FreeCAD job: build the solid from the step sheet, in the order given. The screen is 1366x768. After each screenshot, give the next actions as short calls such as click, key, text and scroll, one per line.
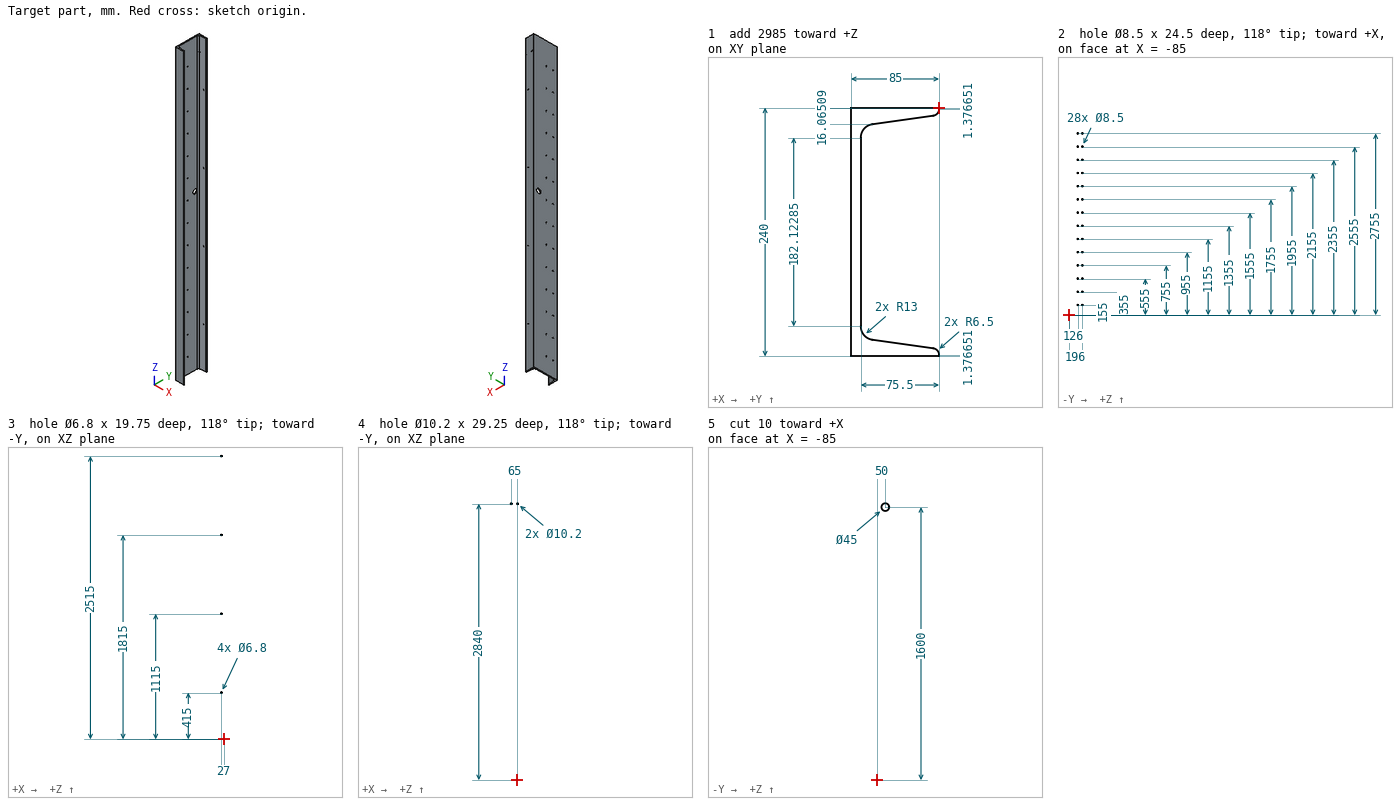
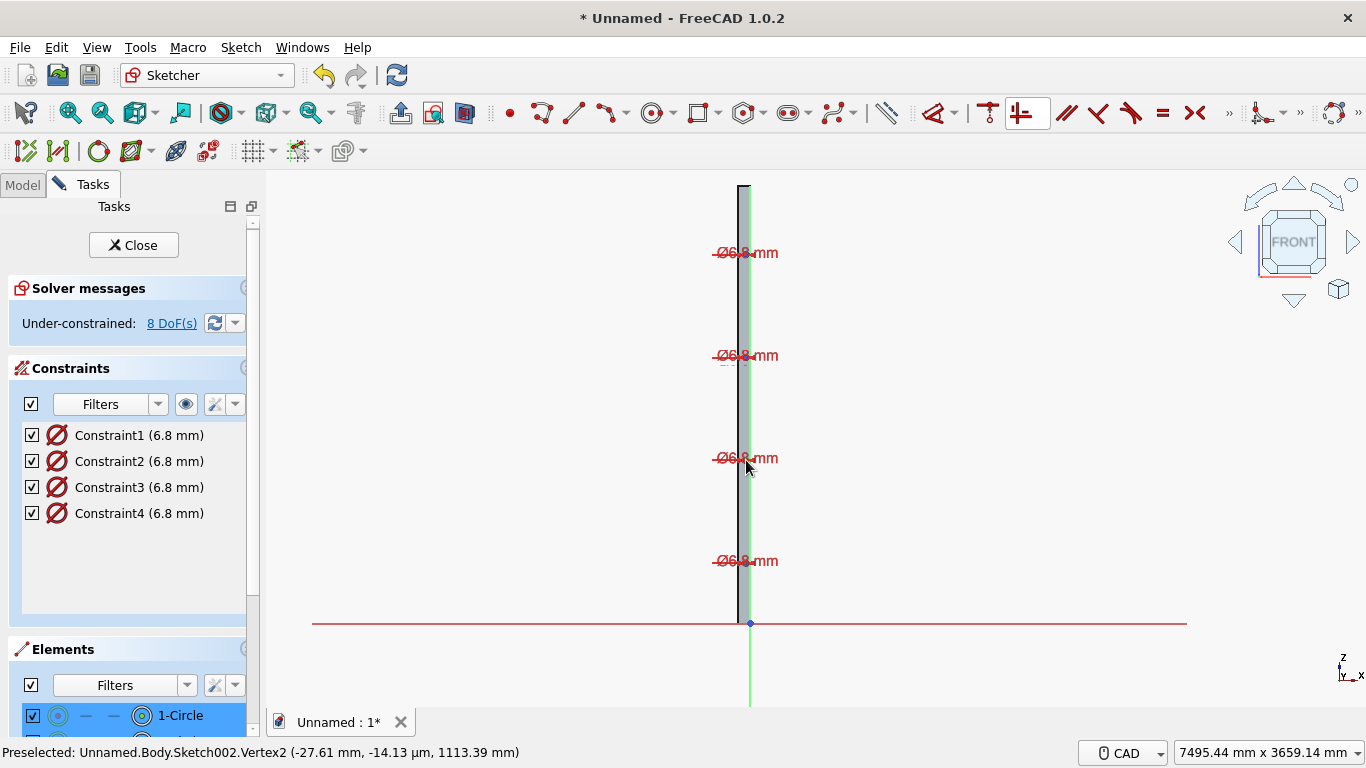
click(1044, 114)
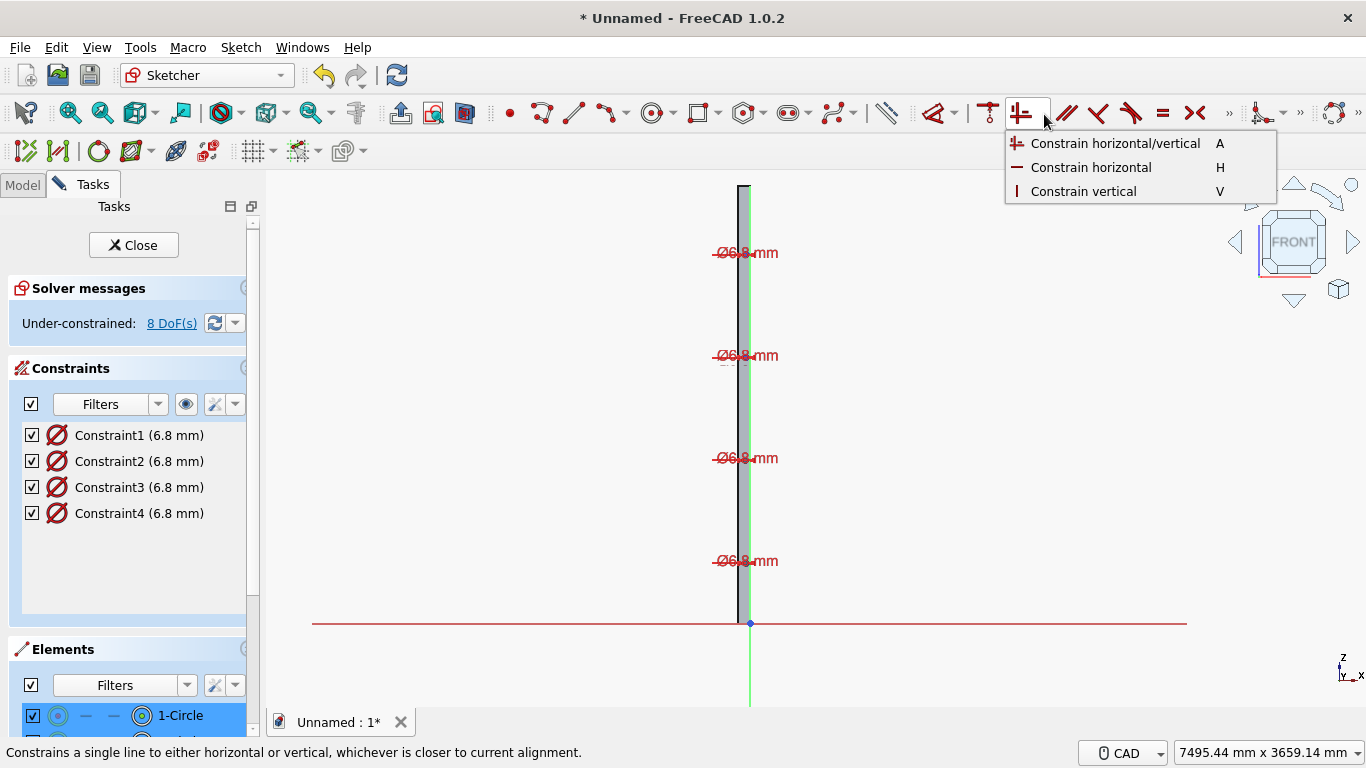
click(1141, 191)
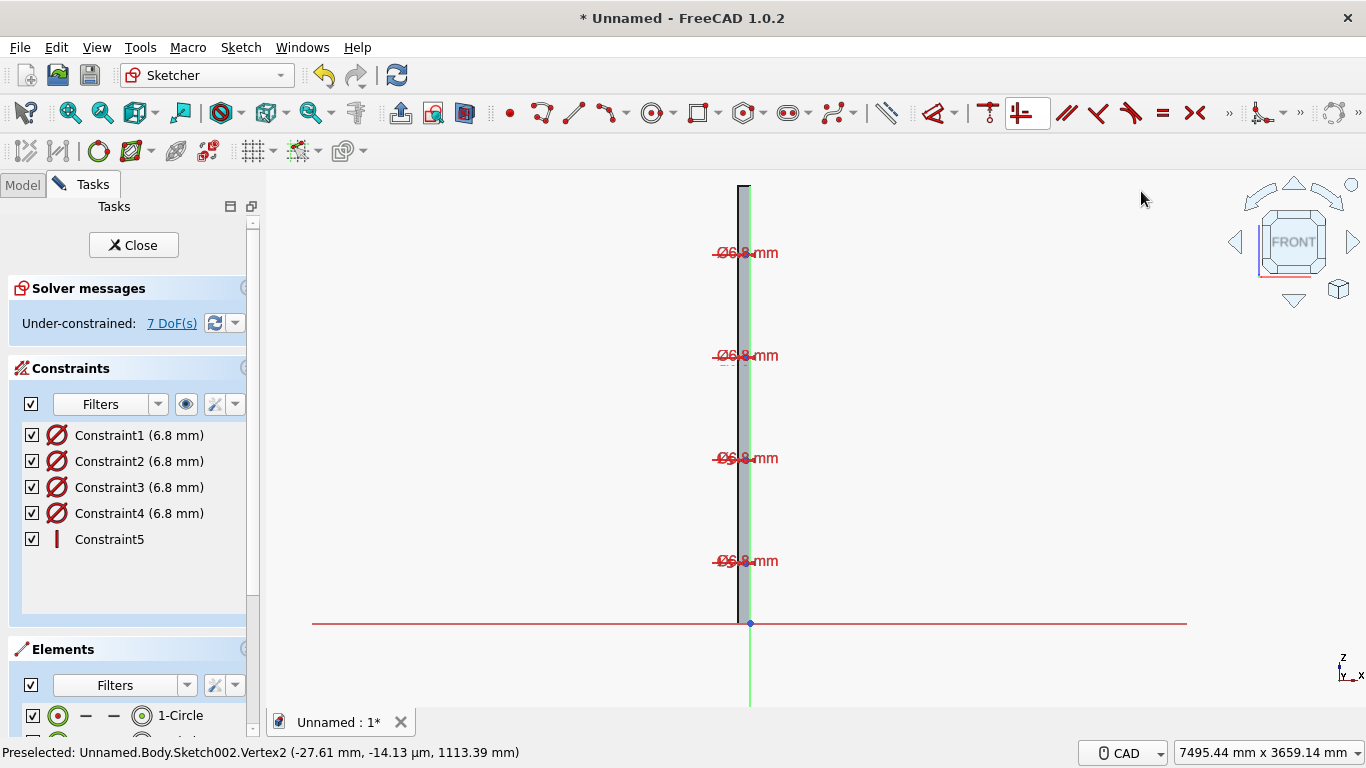
click(746, 460)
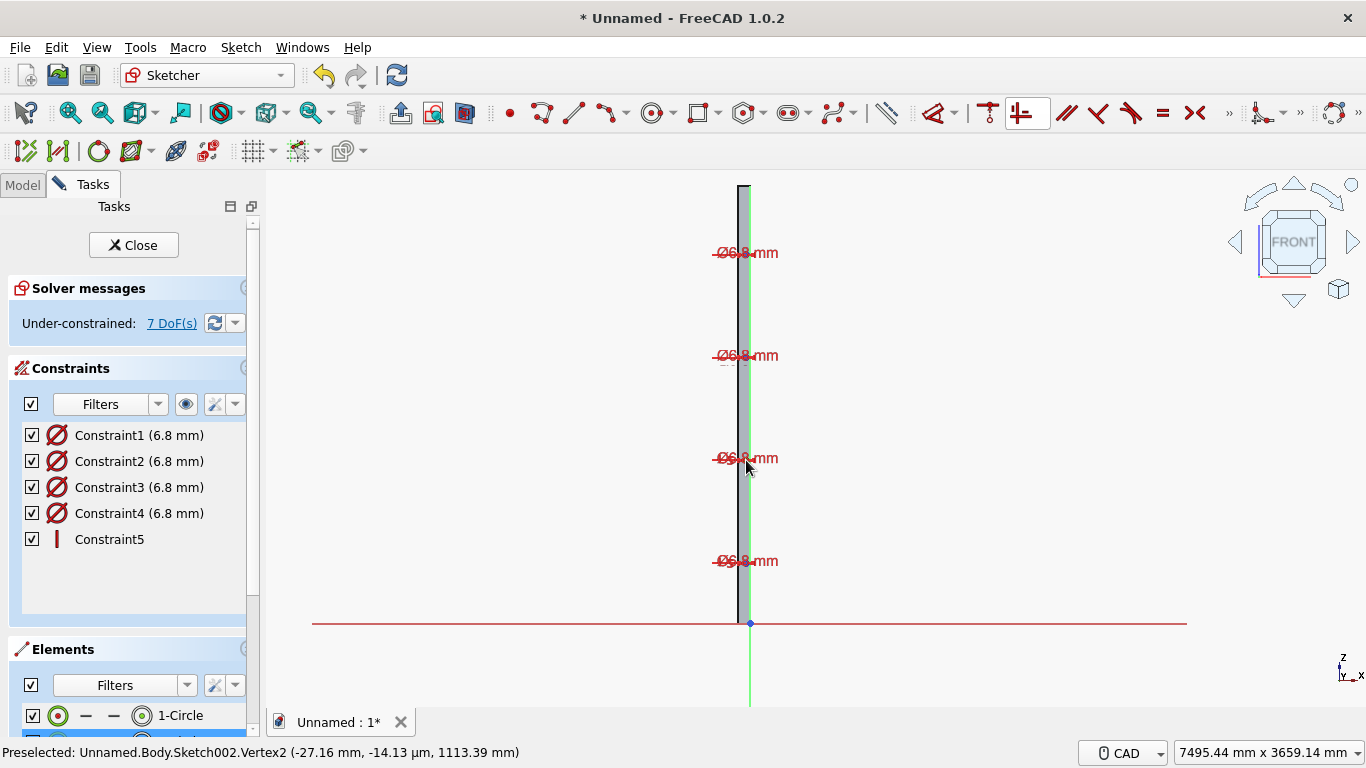
click(746, 358)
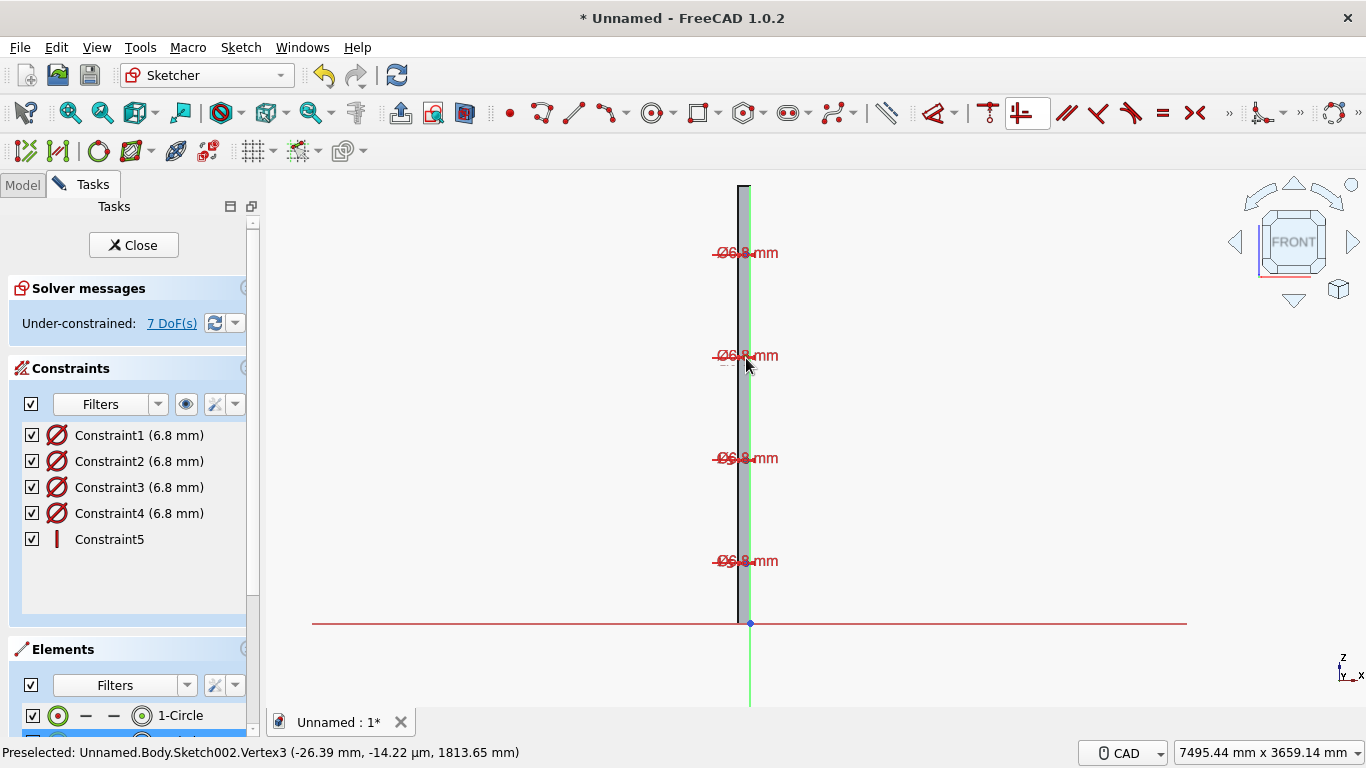
click(1044, 114)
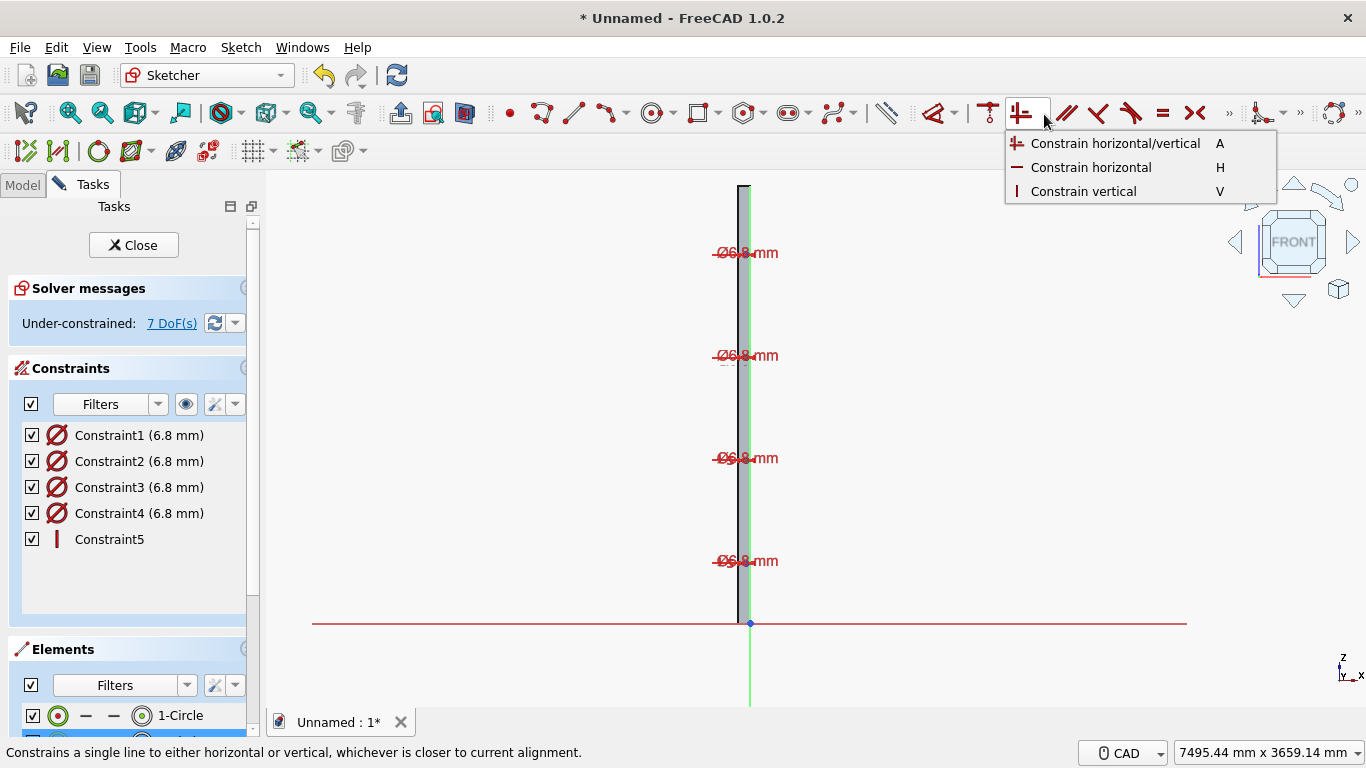
click(1141, 191)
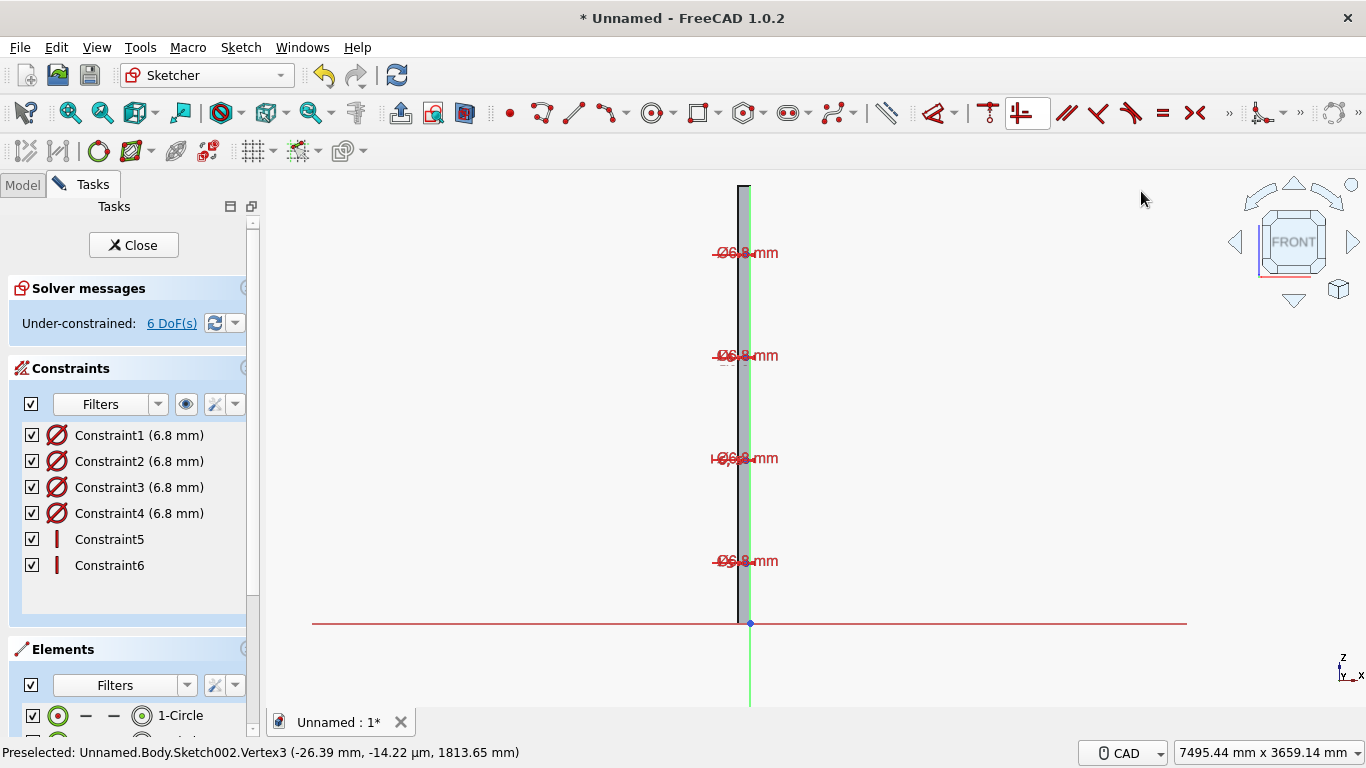
click(746, 358)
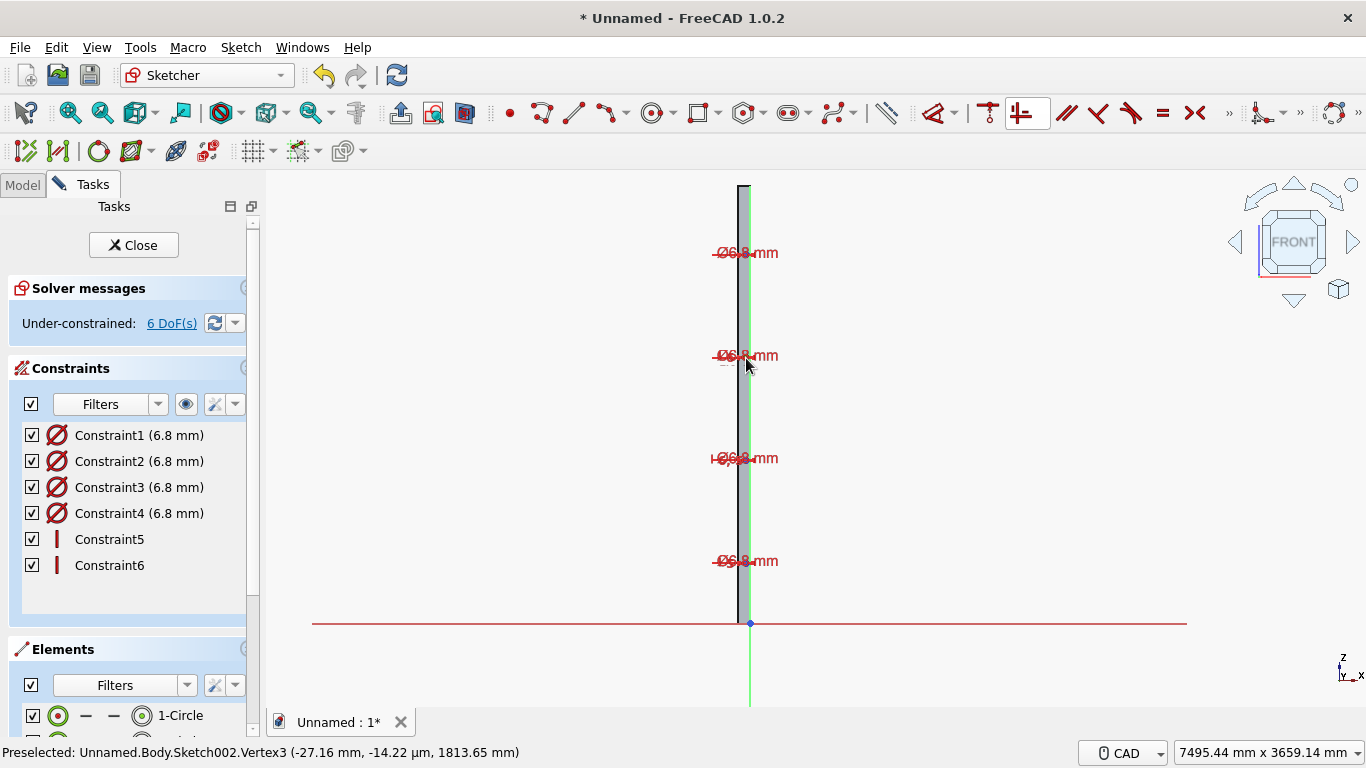
click(746, 255)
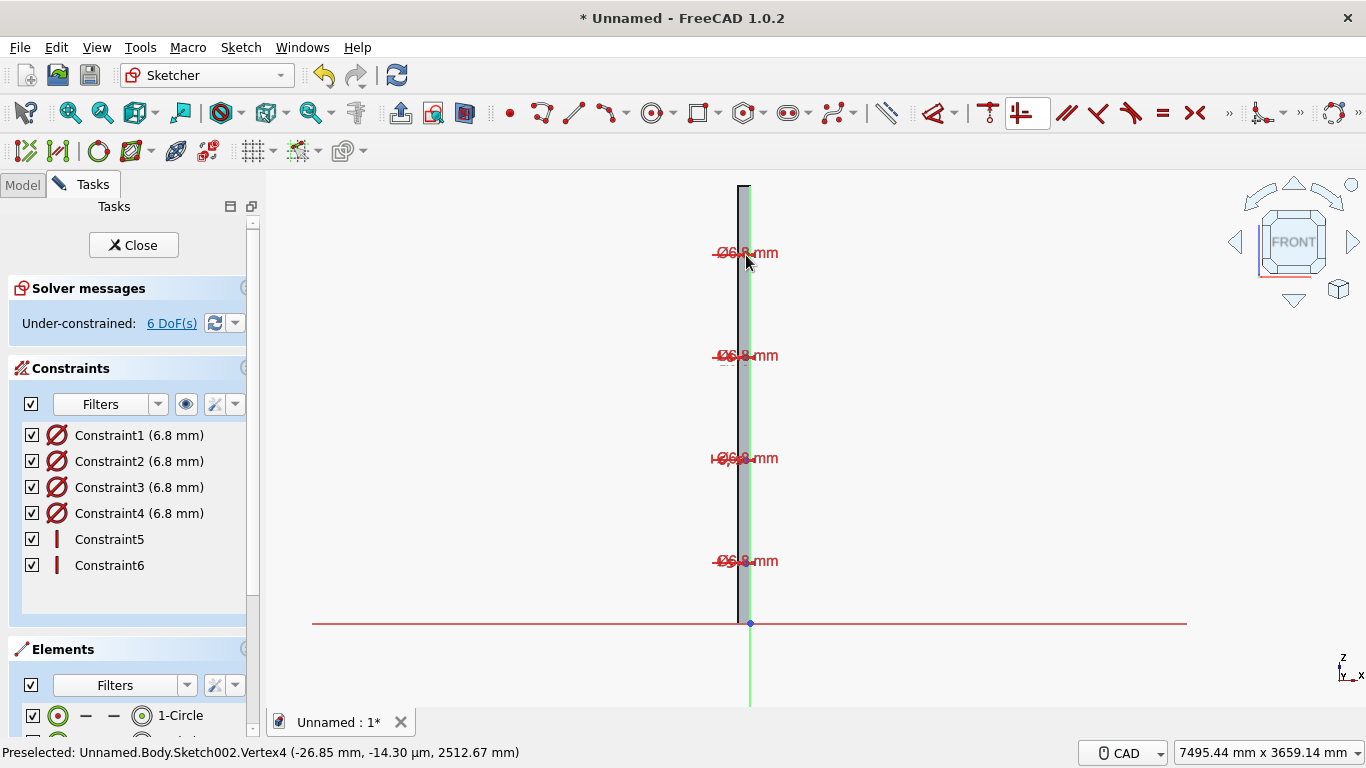
click(1044, 114)